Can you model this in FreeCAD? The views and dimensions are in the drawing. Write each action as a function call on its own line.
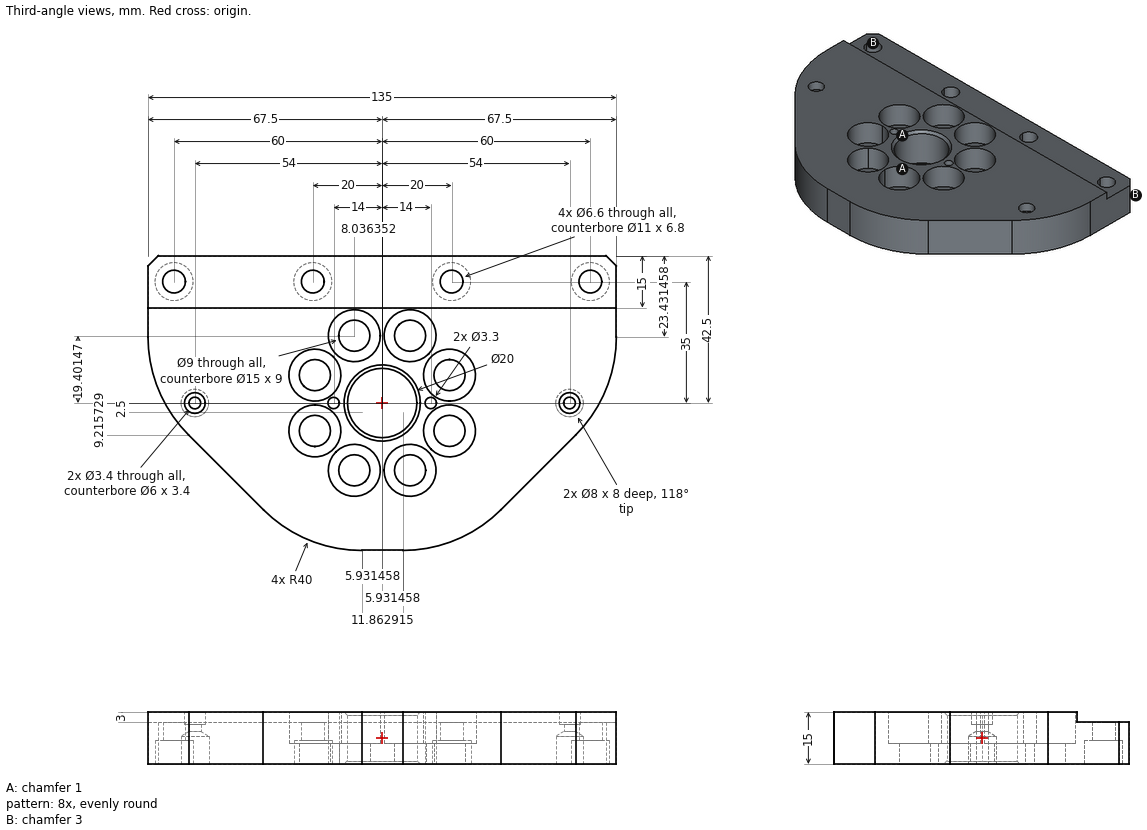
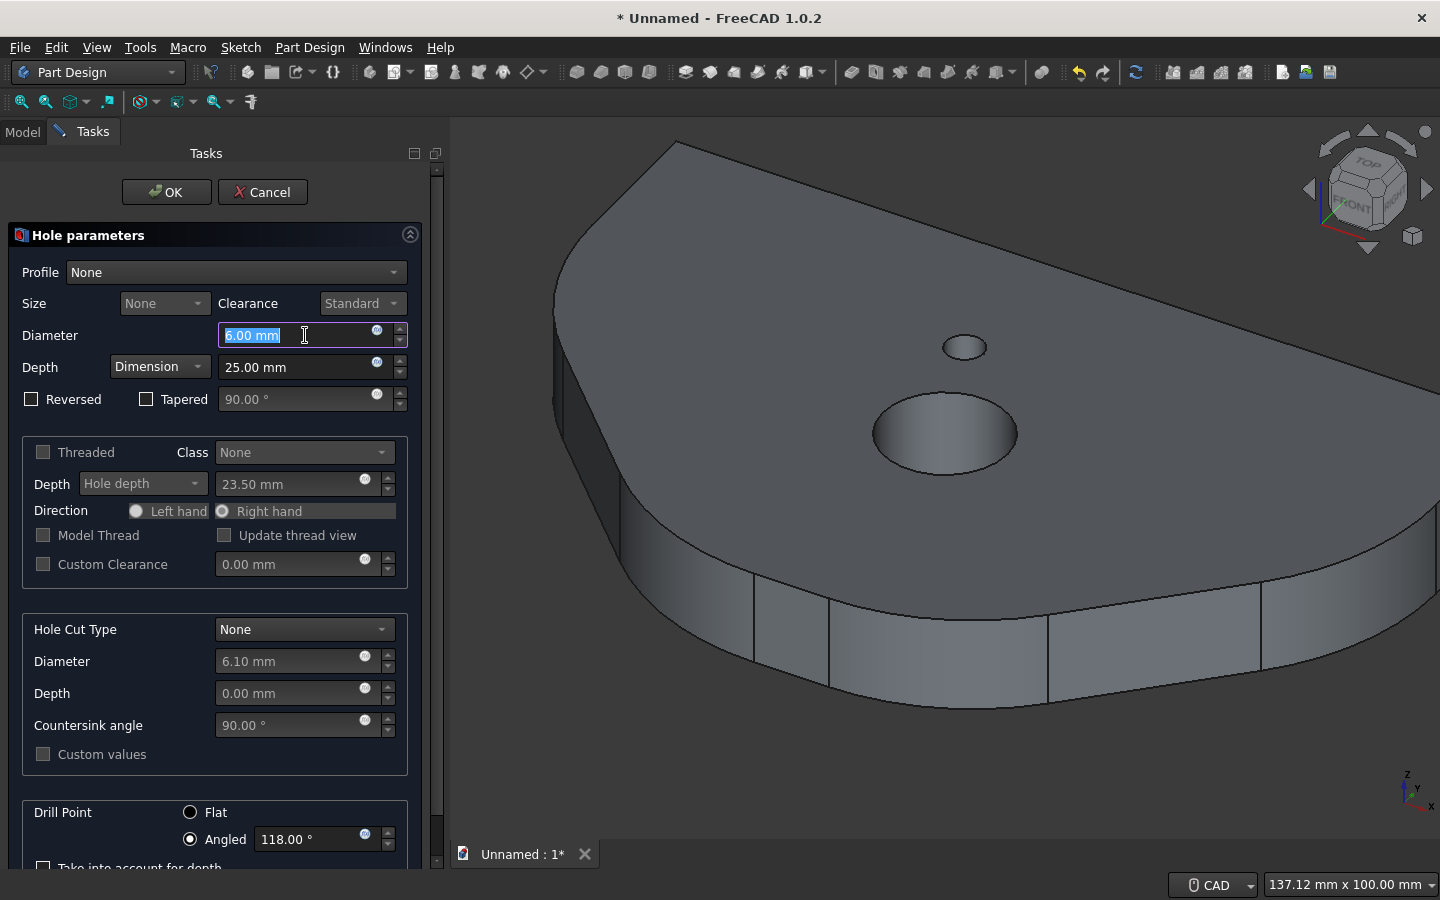
text(9)
key(Tab)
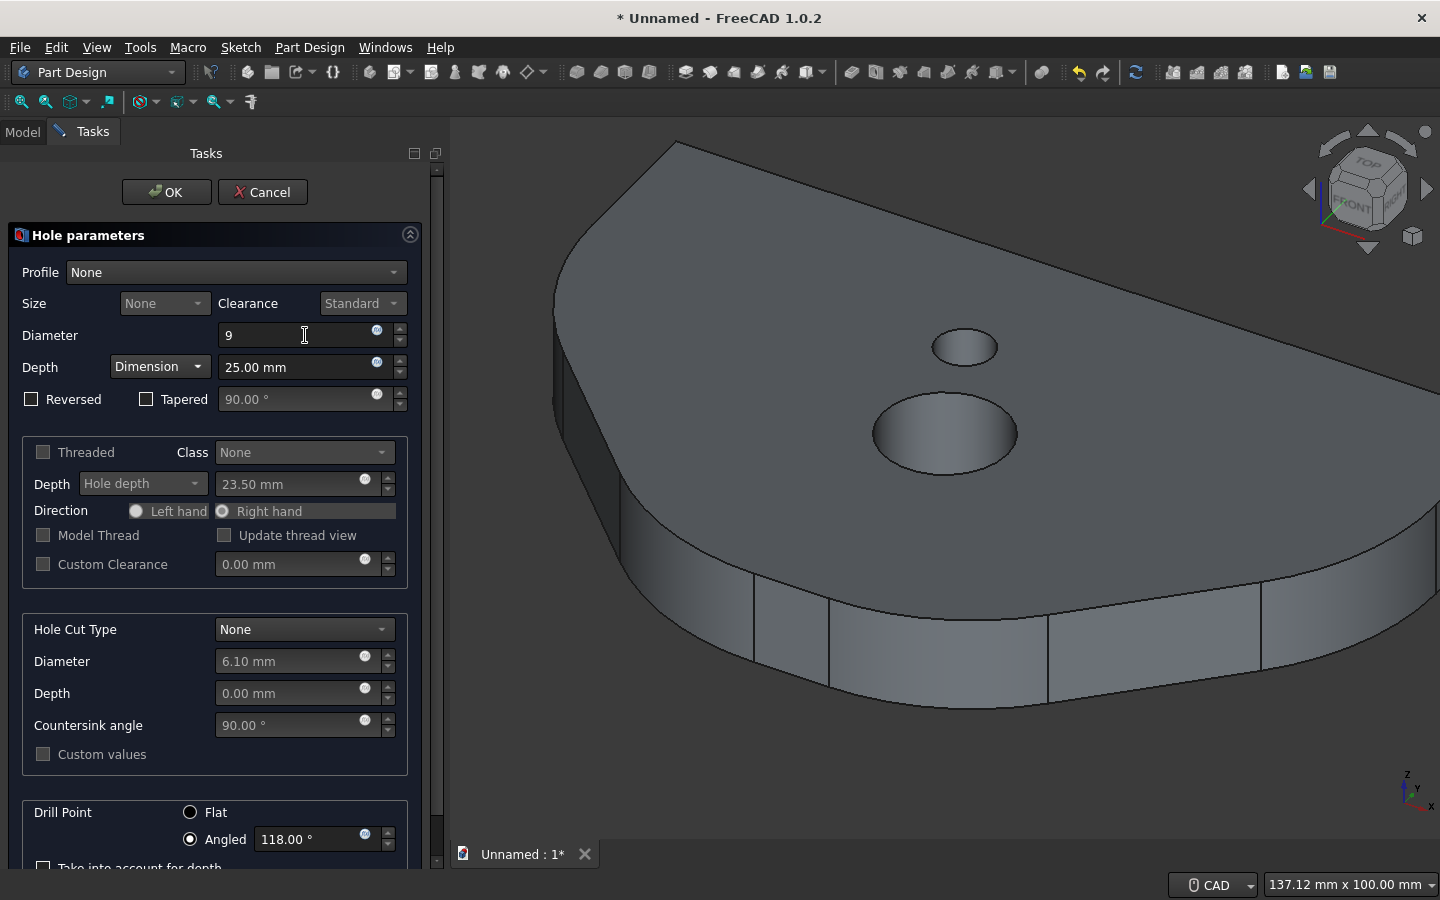
click(161, 366)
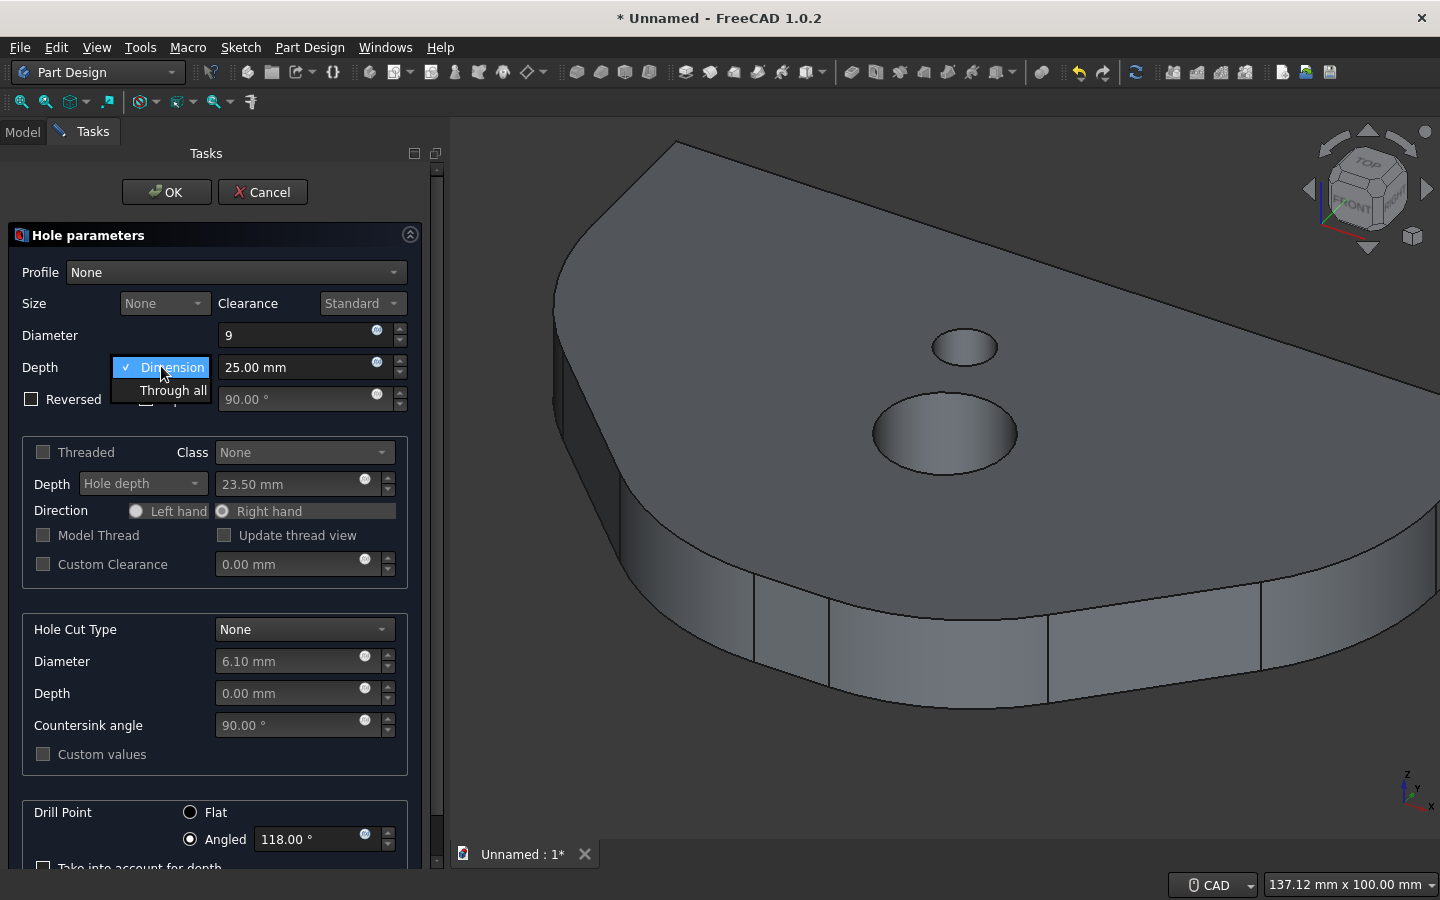
click(160, 390)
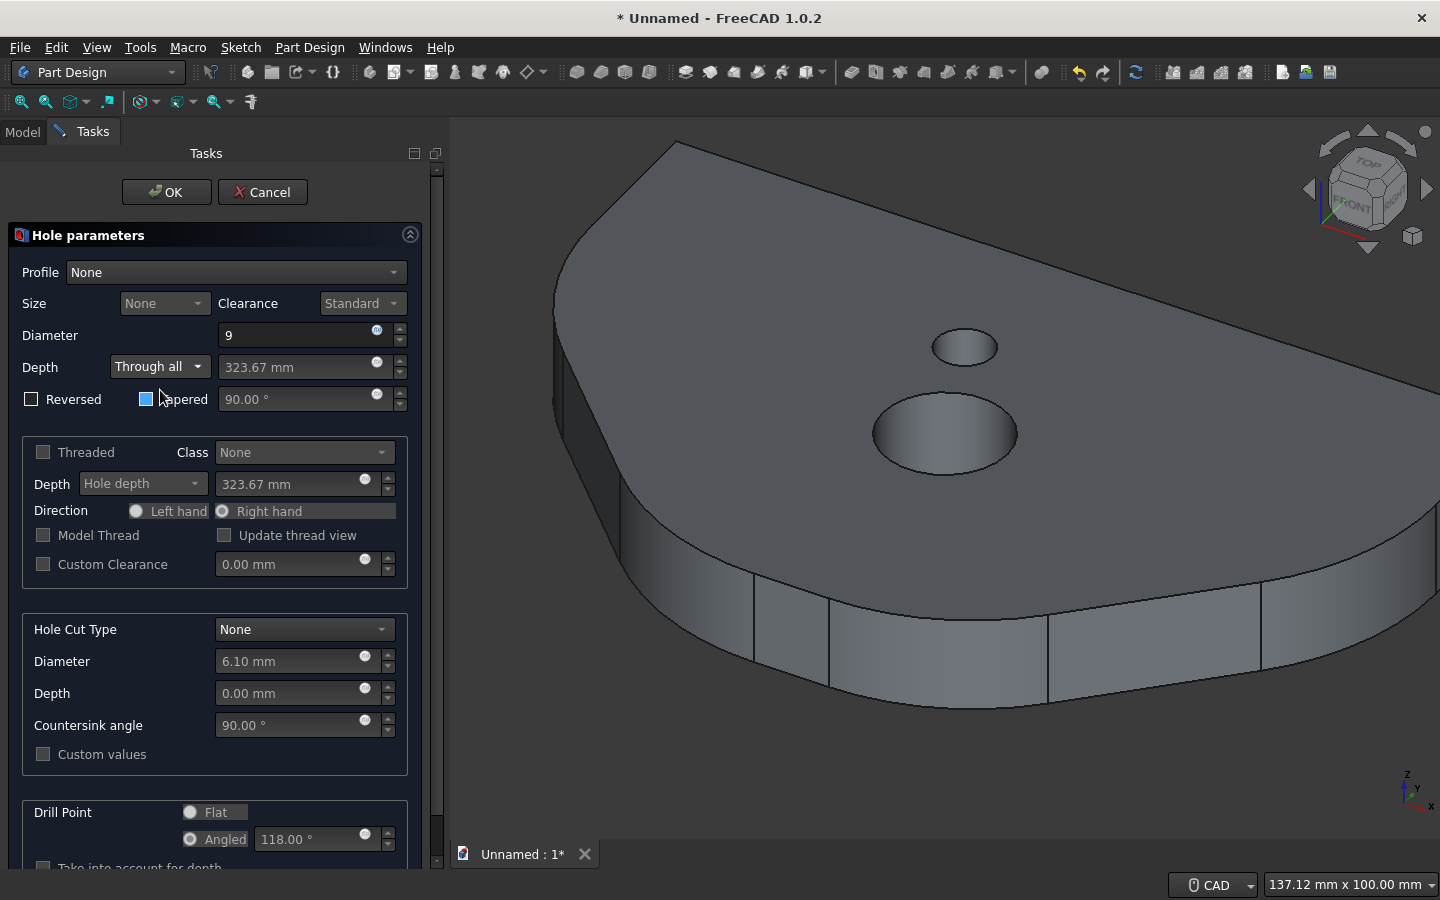
click(306, 630)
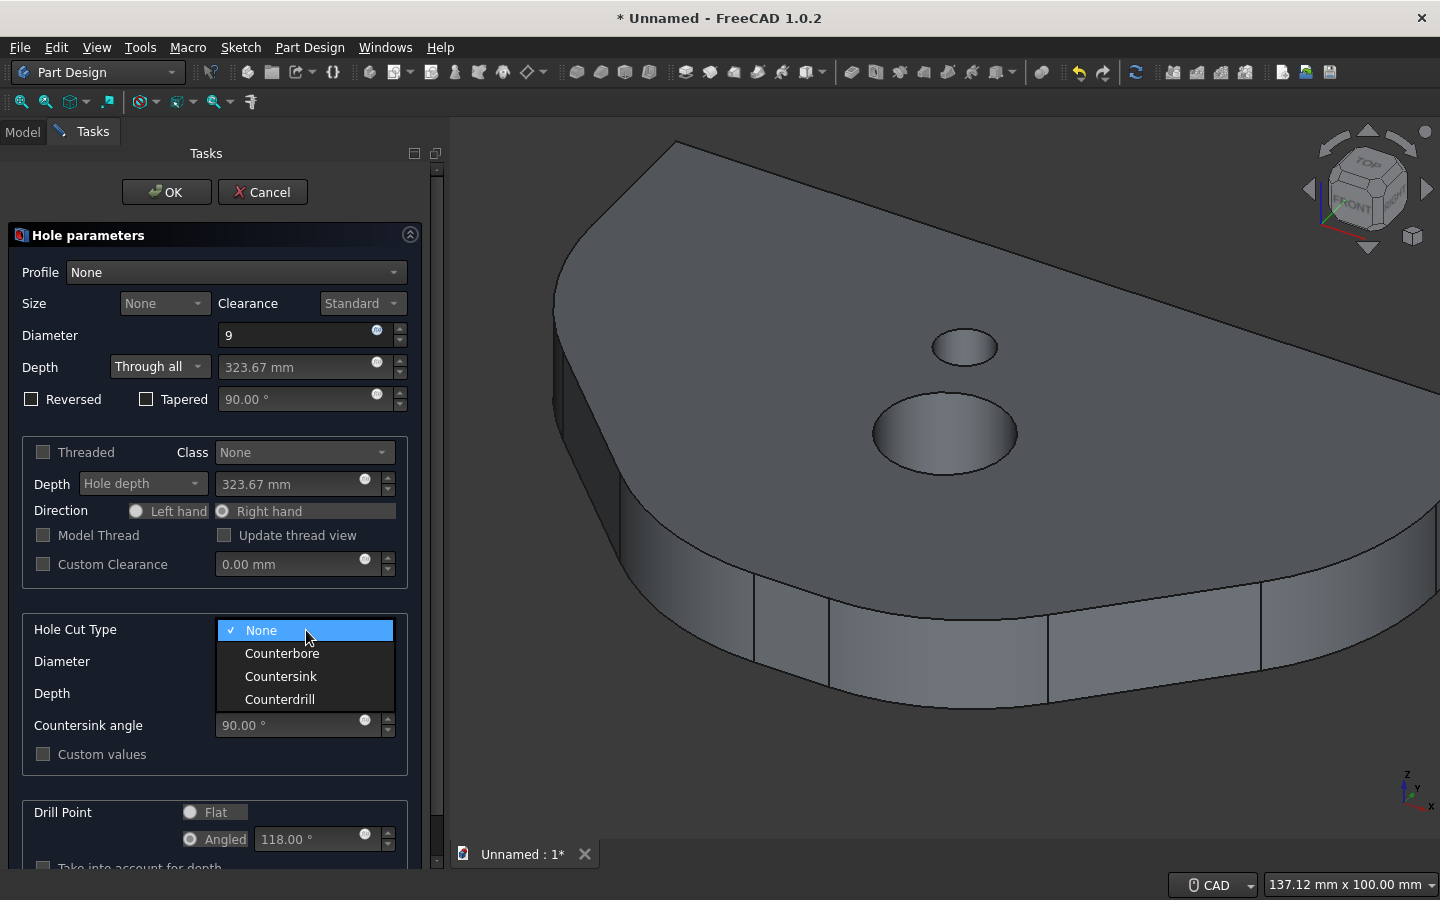
click(304, 654)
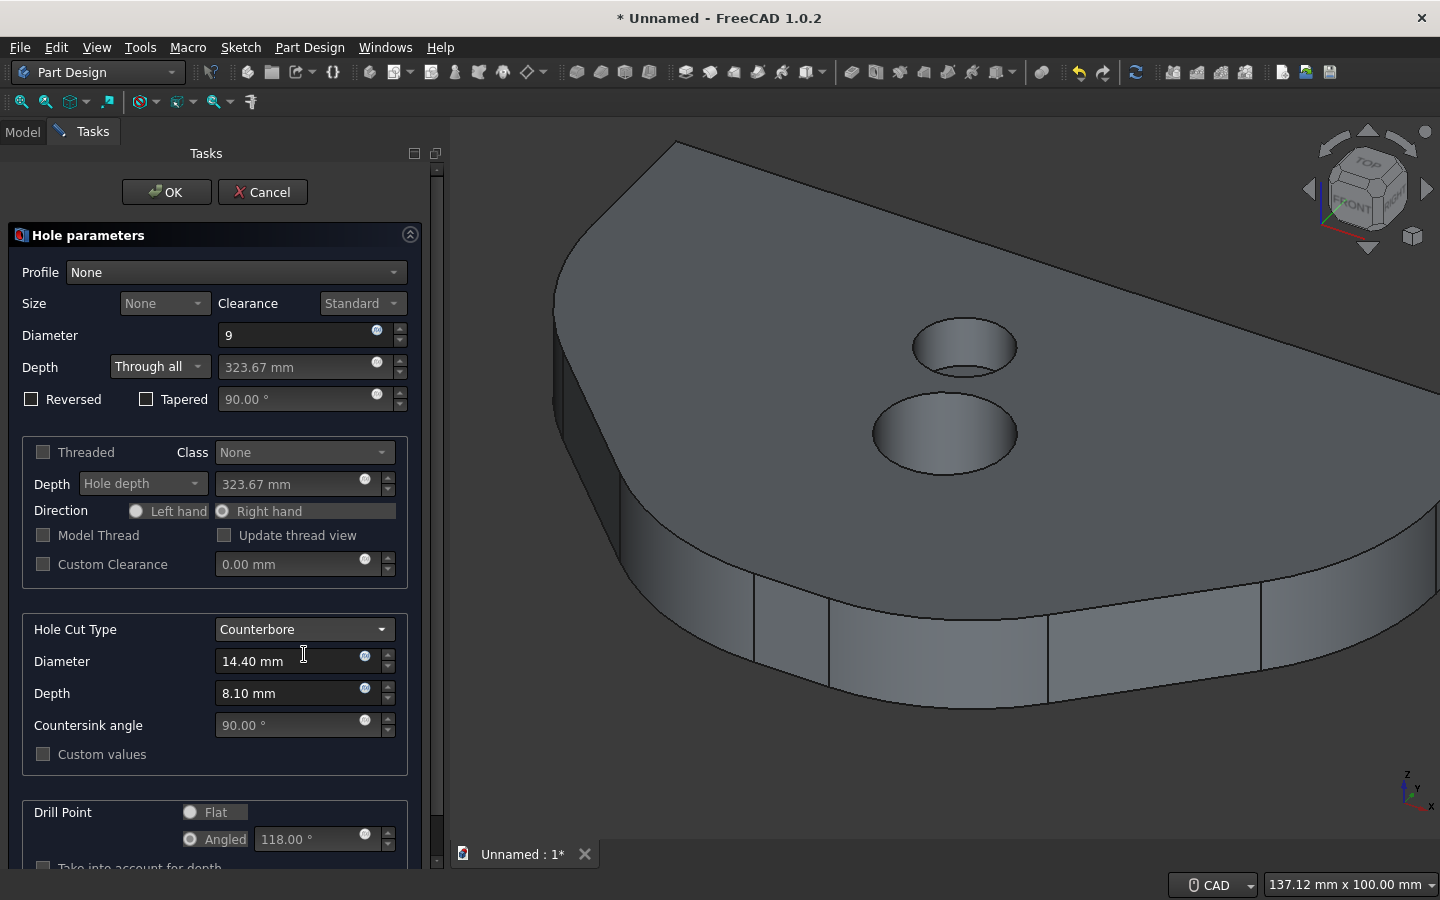
triple_click(298, 661)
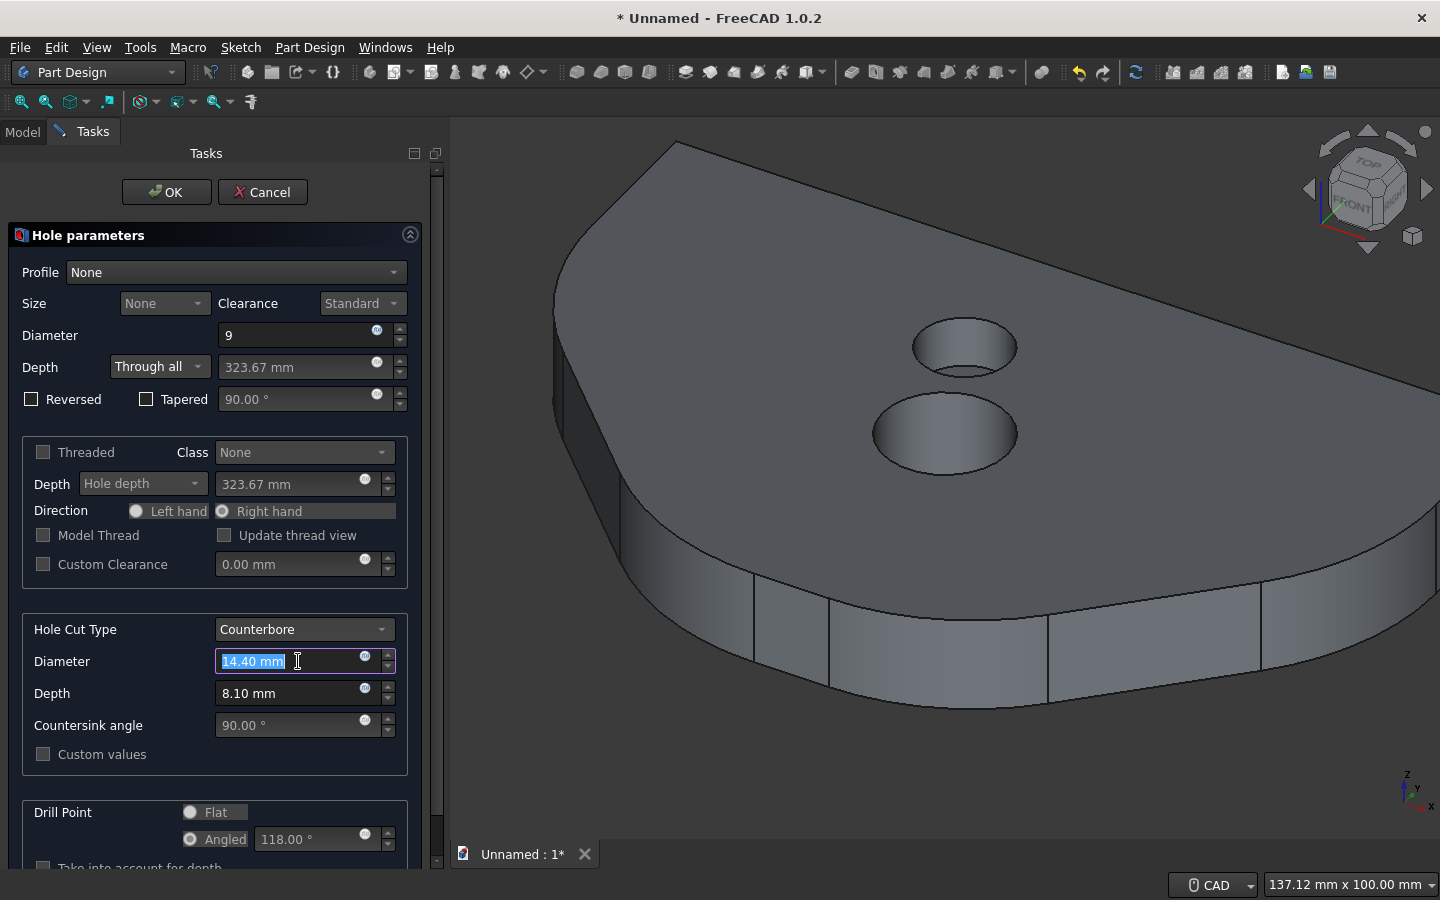
text(15)
key(Tab)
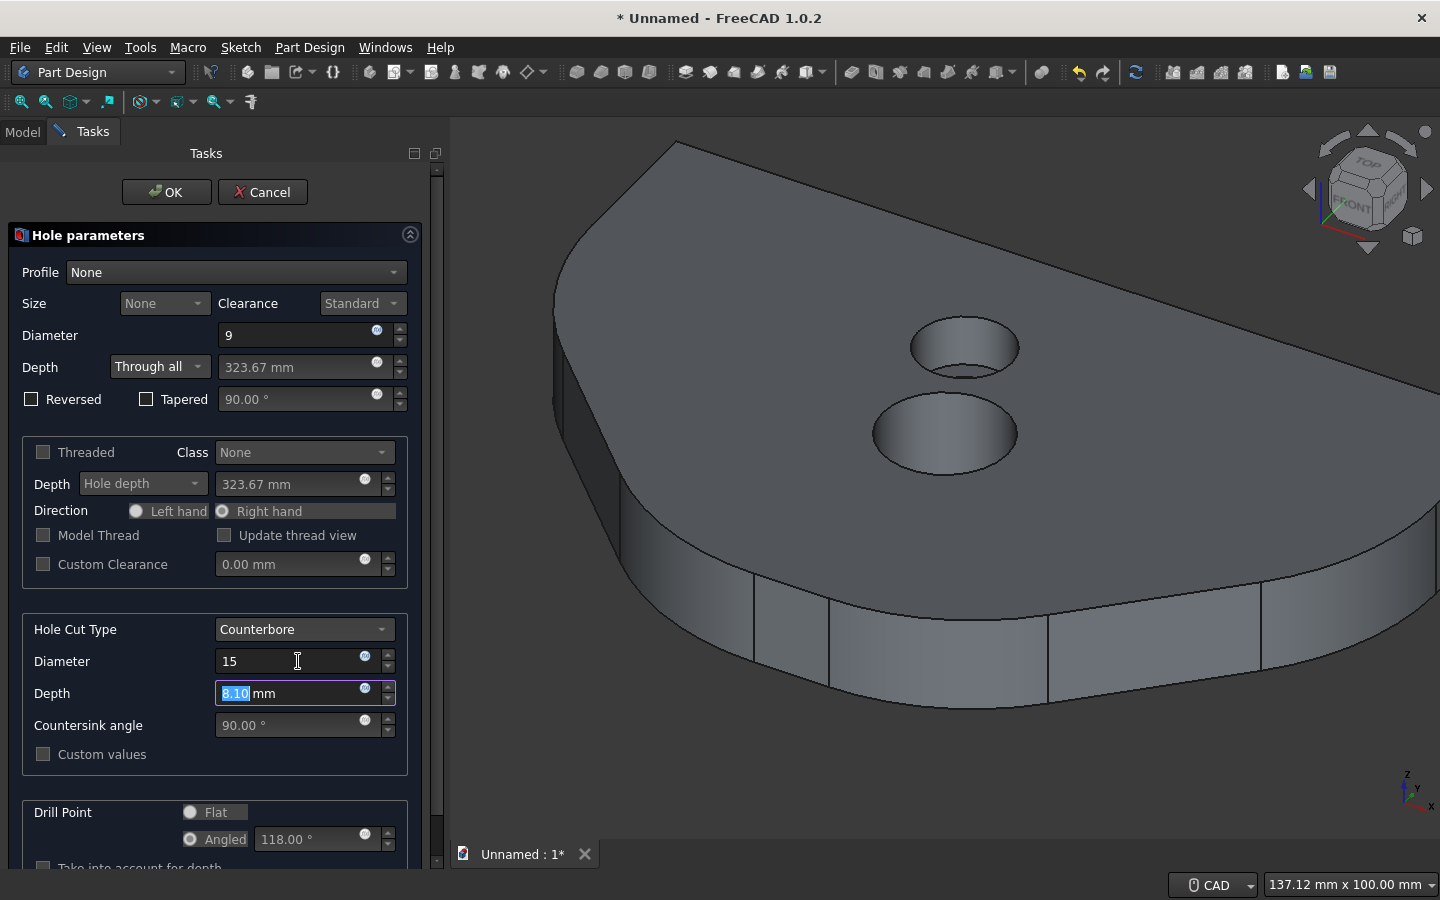
text(9)
key(Tab)